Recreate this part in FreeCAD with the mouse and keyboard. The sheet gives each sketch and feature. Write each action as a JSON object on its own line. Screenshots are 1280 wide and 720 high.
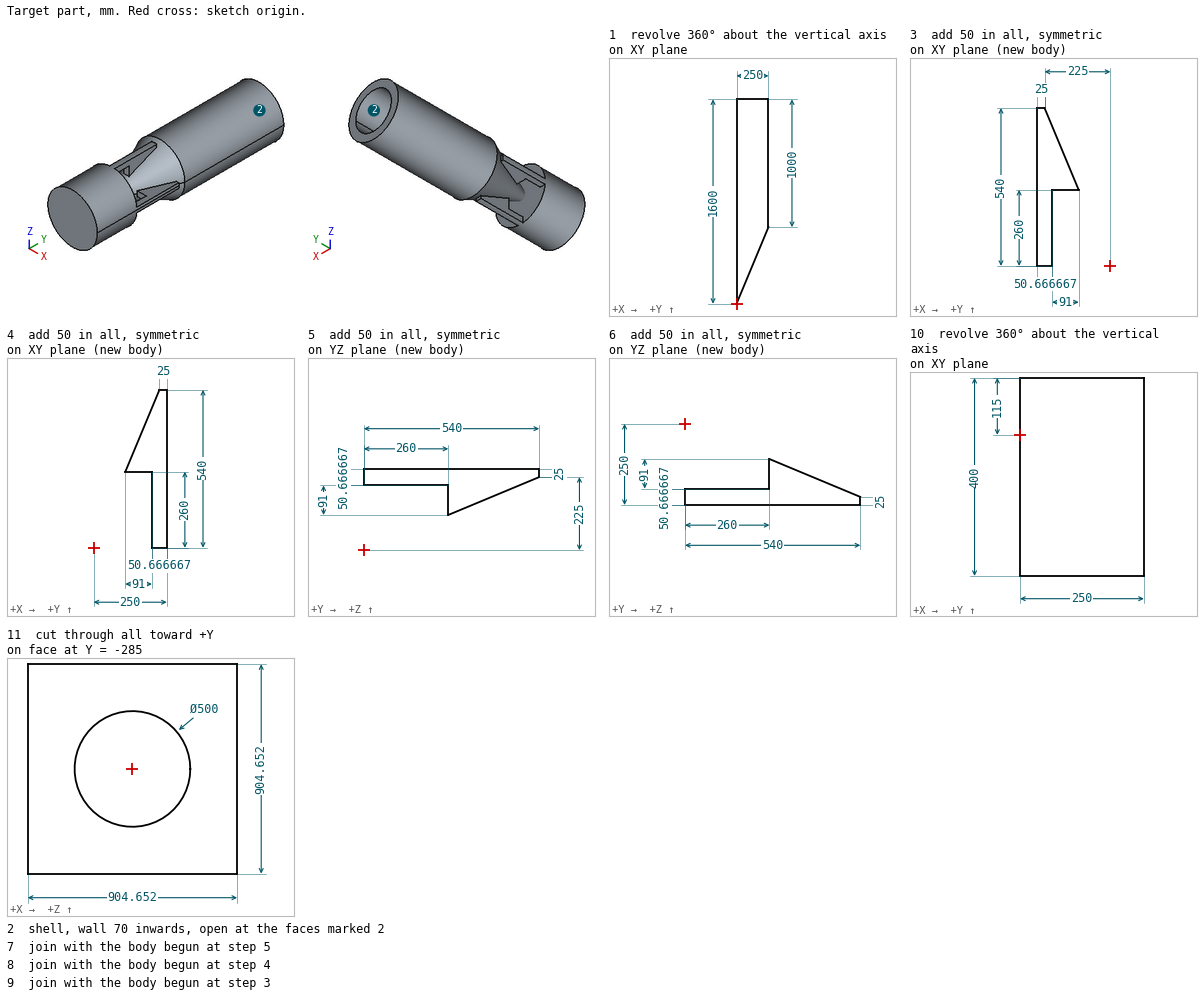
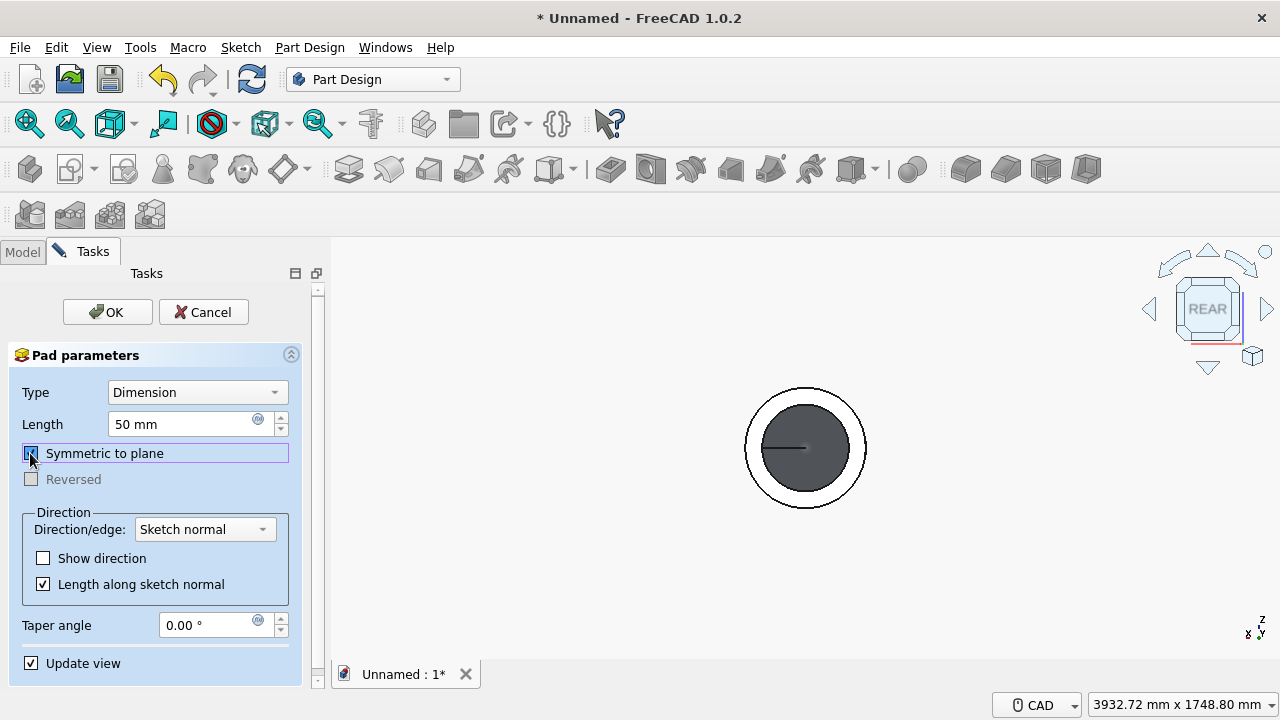
{"action": "left_click", "coordinate": [108, 312]}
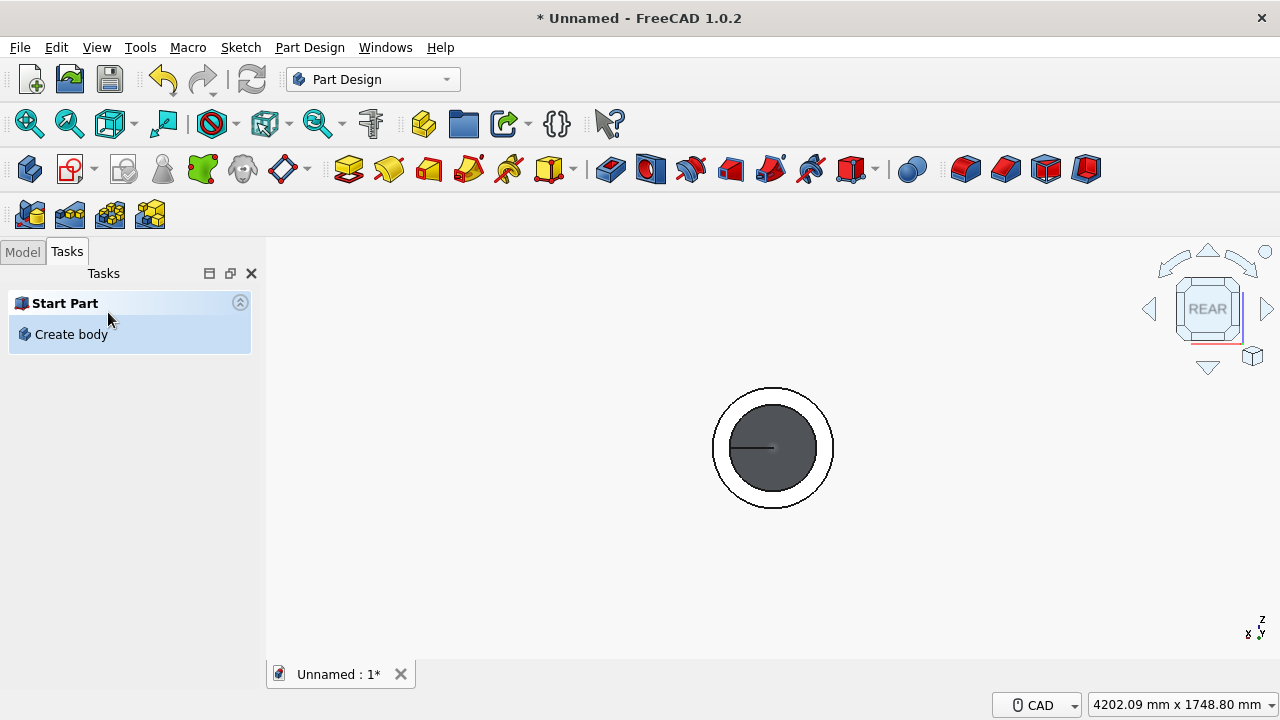
{"action": "left_click", "coordinate": [30, 124]}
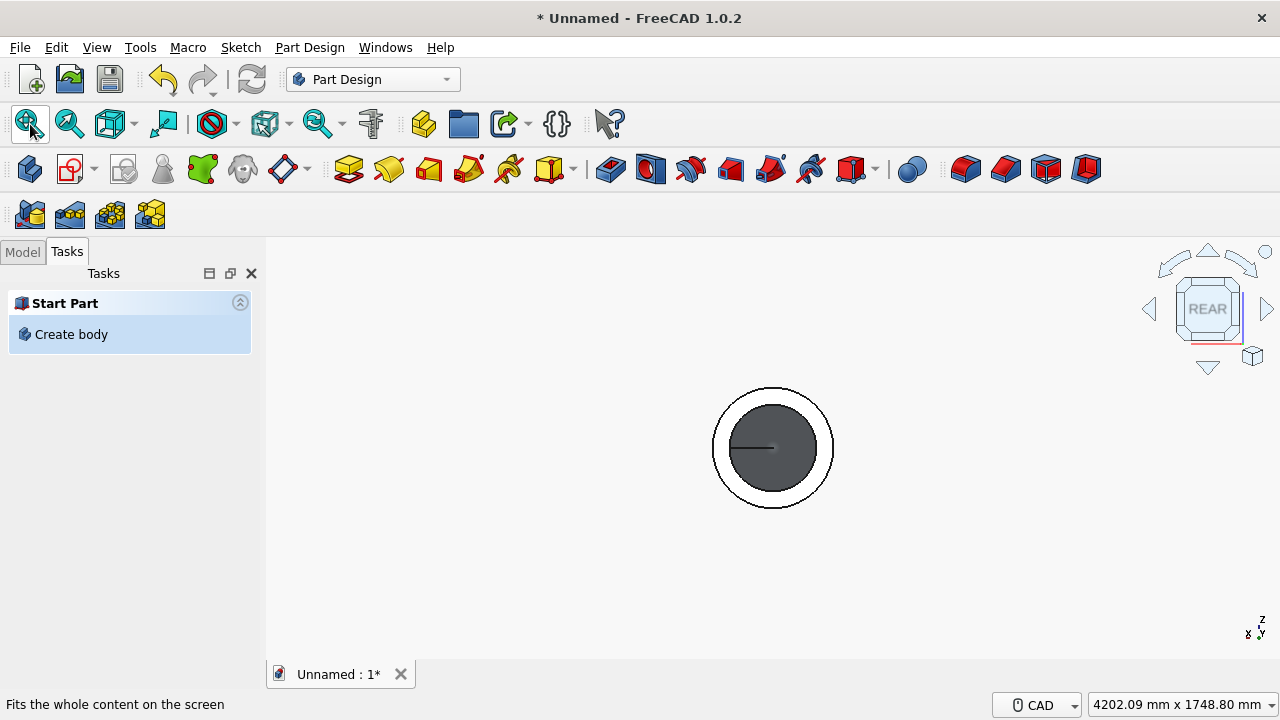
{"action": "left_click", "coordinate": [30, 170]}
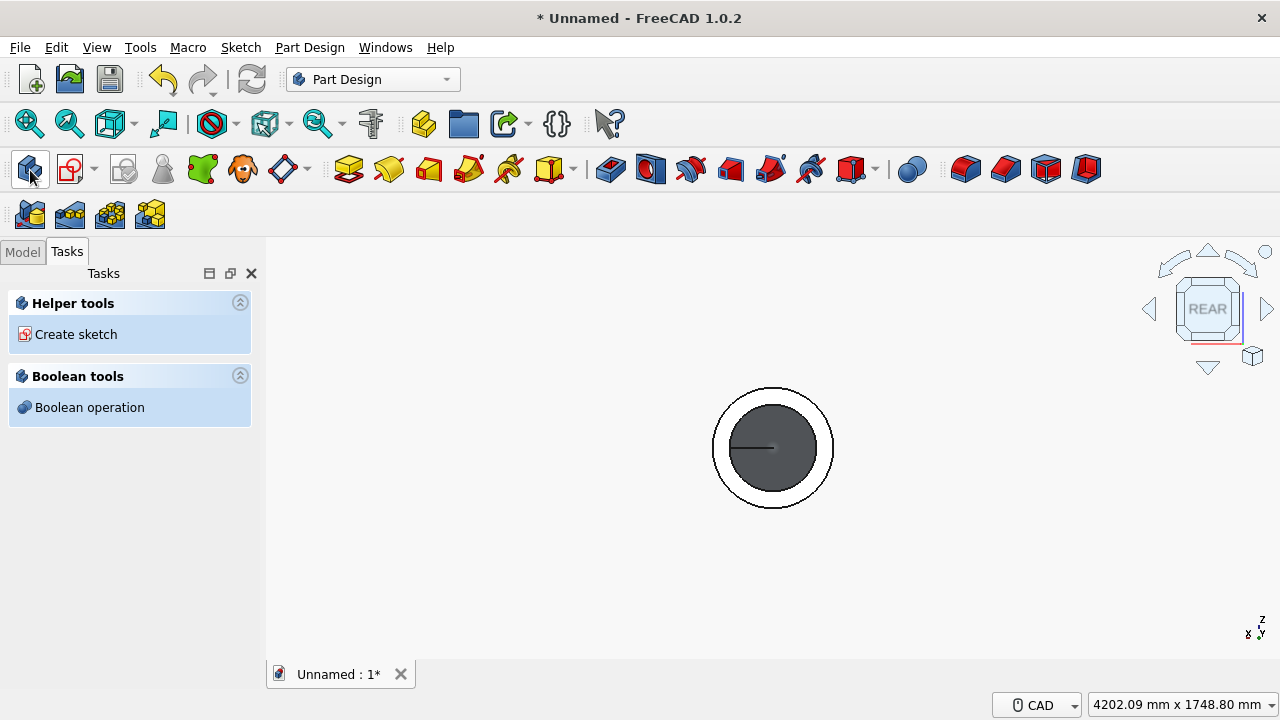
{"action": "left_click", "coordinate": [306, 619]}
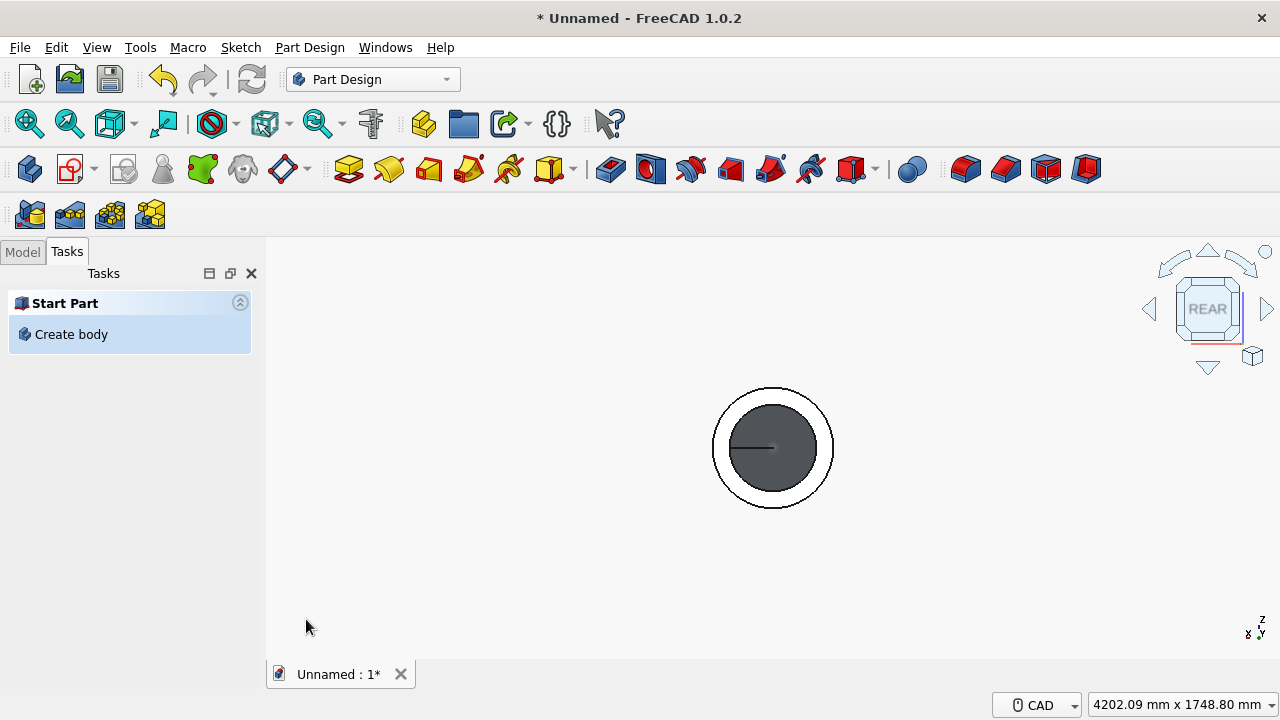
{"action": "left_click", "coordinate": [70, 170]}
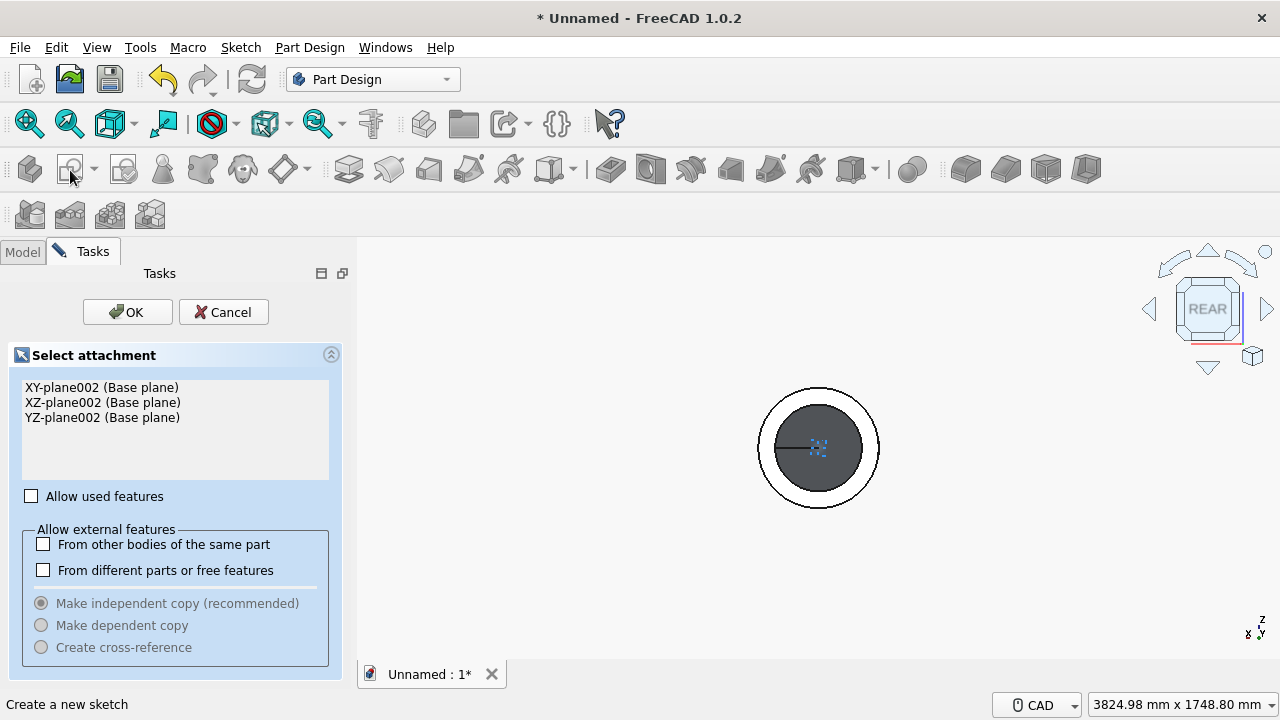
{"action": "left_click", "coordinate": [82, 388]}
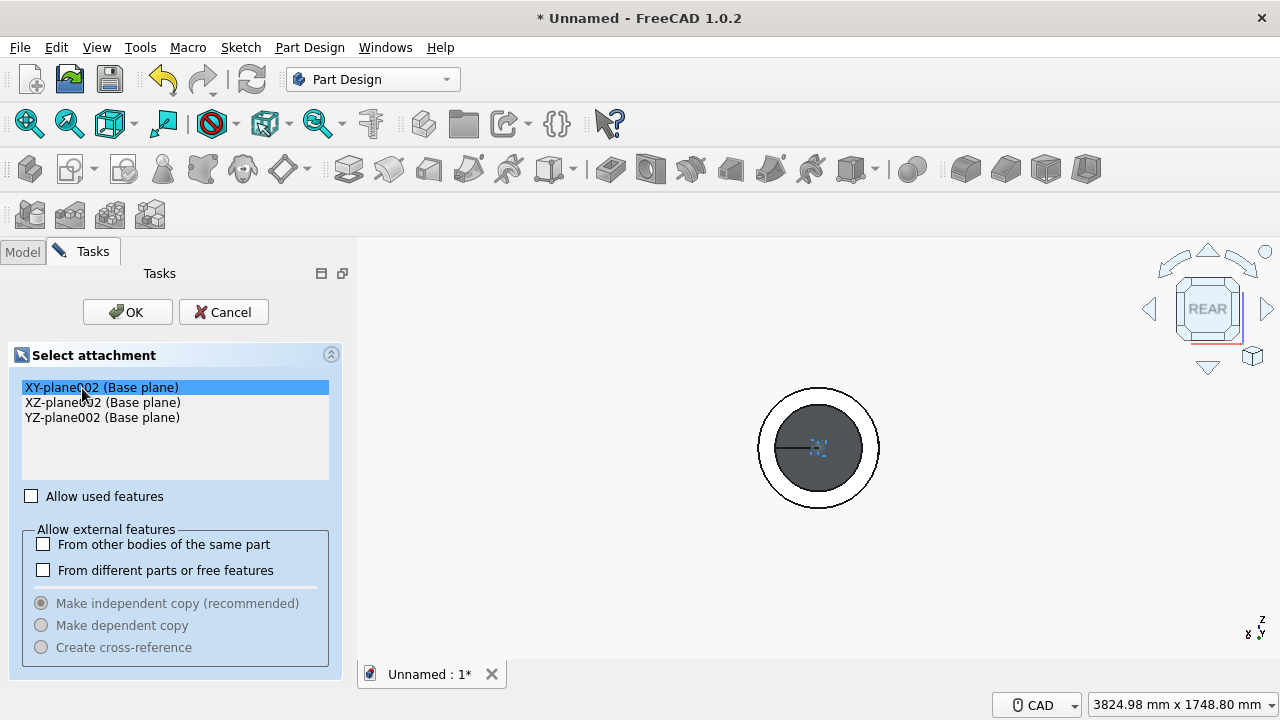
{"action": "left_click", "coordinate": [128, 312]}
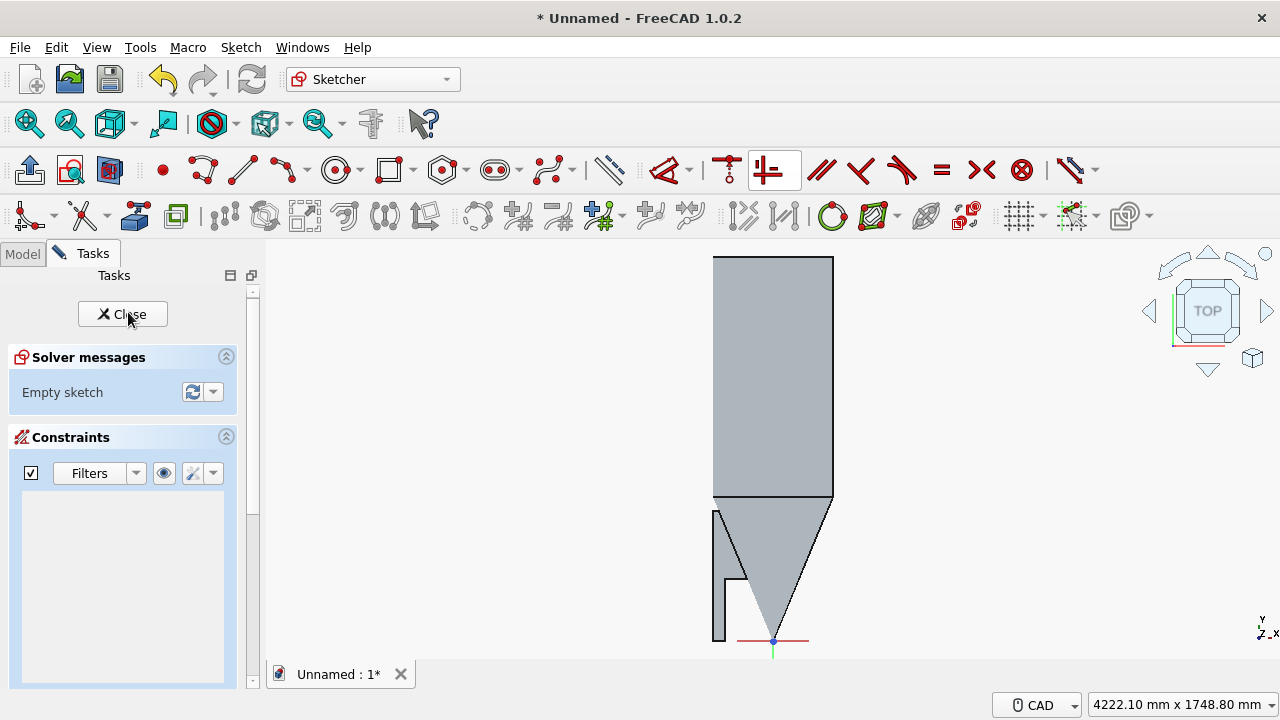
{"action": "scroll", "coordinate": [704, 449], "scroll_direction": "down", "scroll_amount": 5}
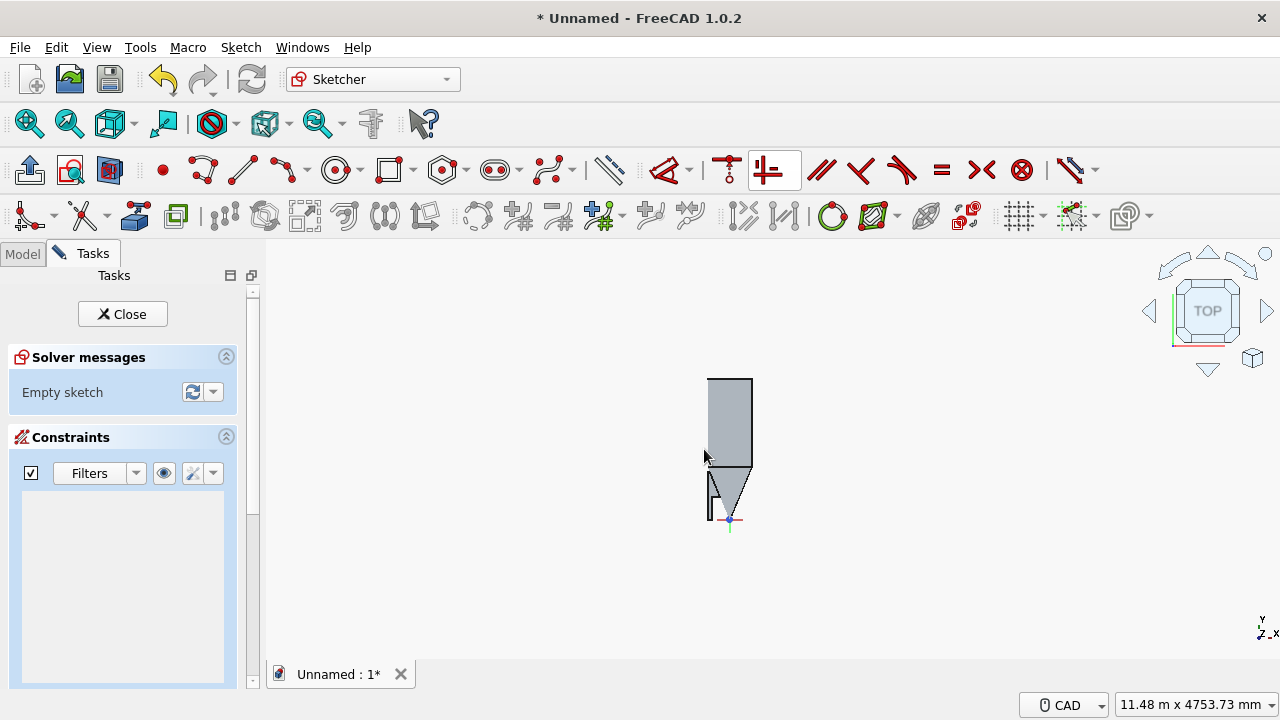
{"action": "scroll", "coordinate": [750, 508], "scroll_direction": "up", "scroll_amount": 8}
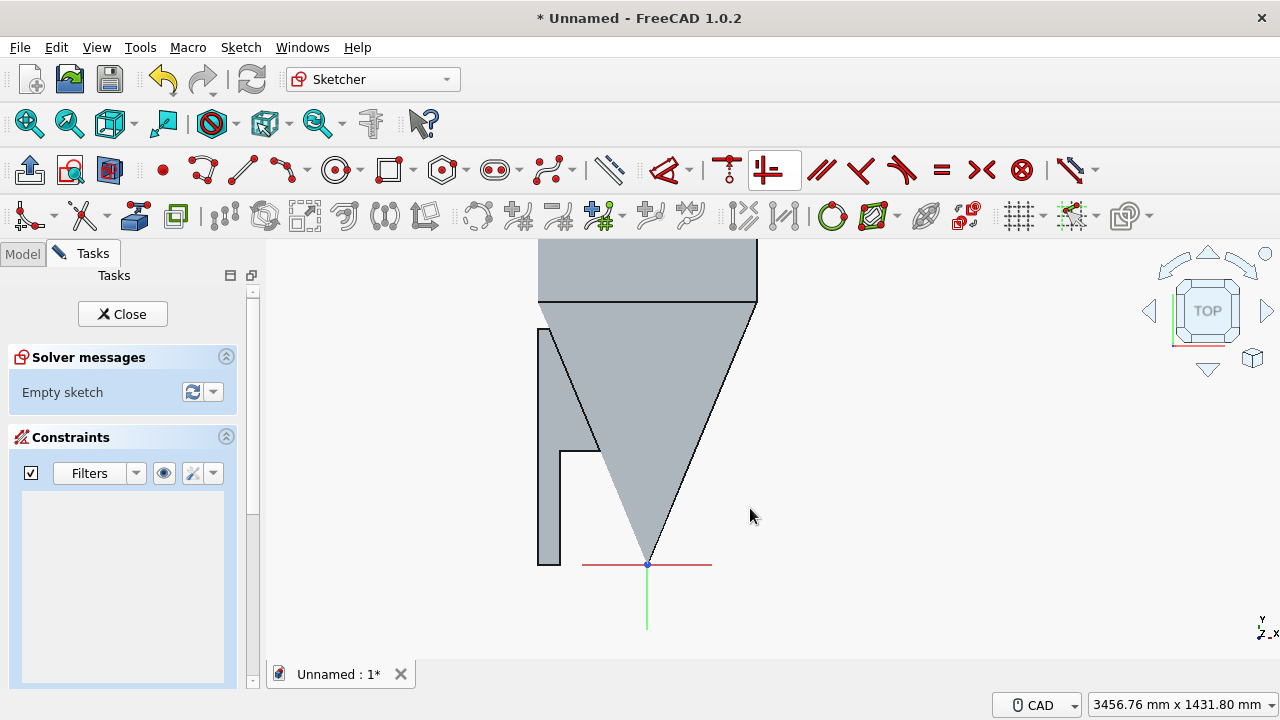
{"action": "left_click", "coordinate": [204, 170]}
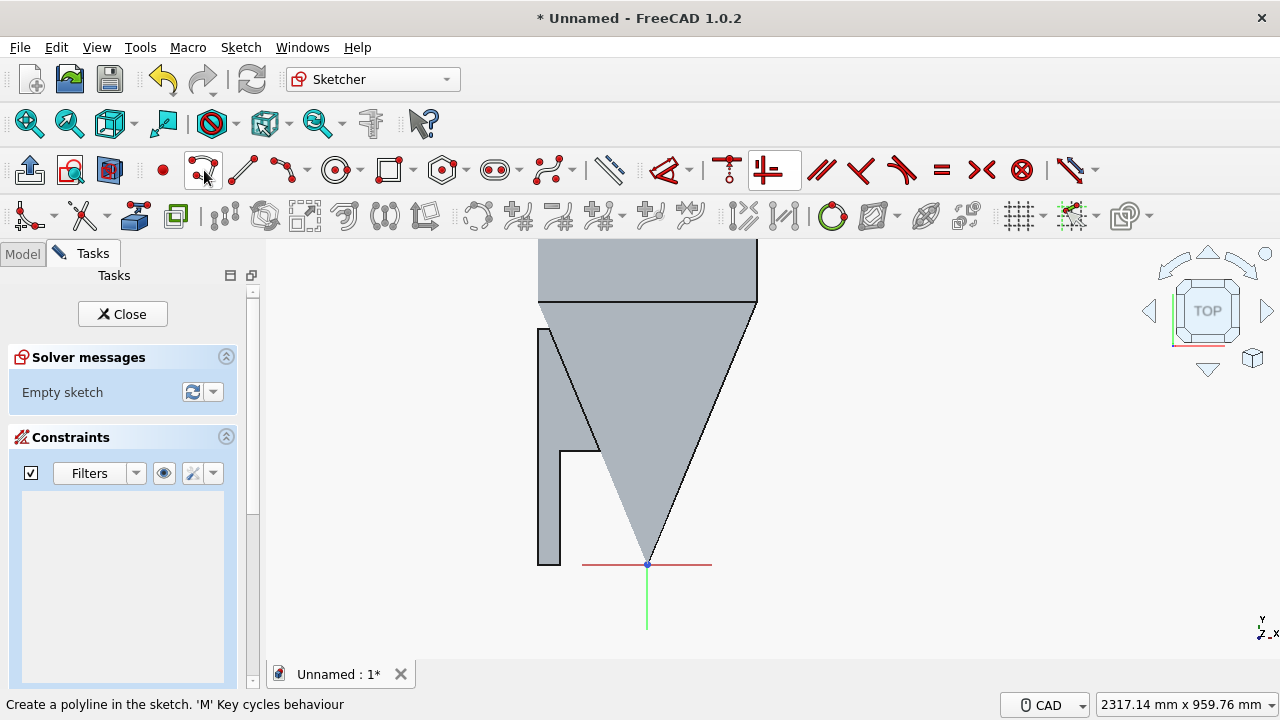
{"action": "left_click", "coordinate": [735, 565]}
{"action": "left_click", "coordinate": [757, 556]}
{"action": "left_click", "coordinate": [757, 329]}